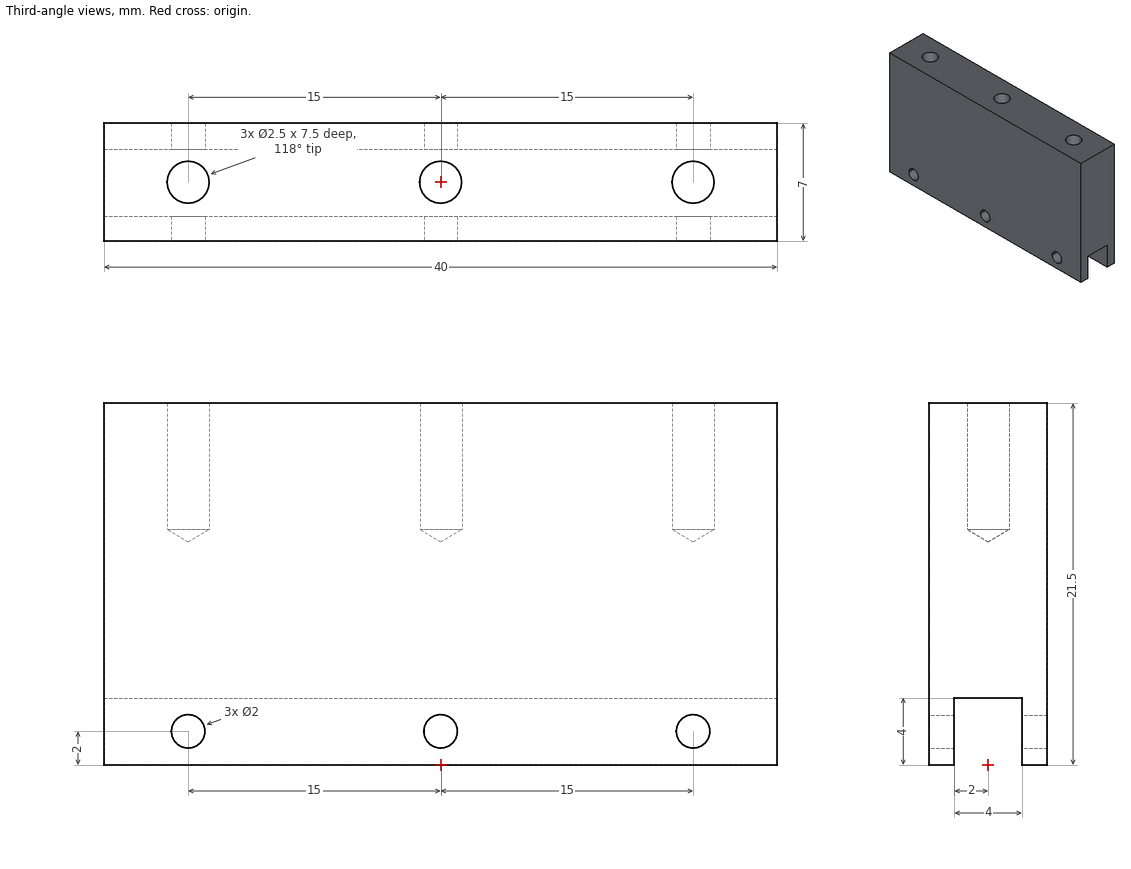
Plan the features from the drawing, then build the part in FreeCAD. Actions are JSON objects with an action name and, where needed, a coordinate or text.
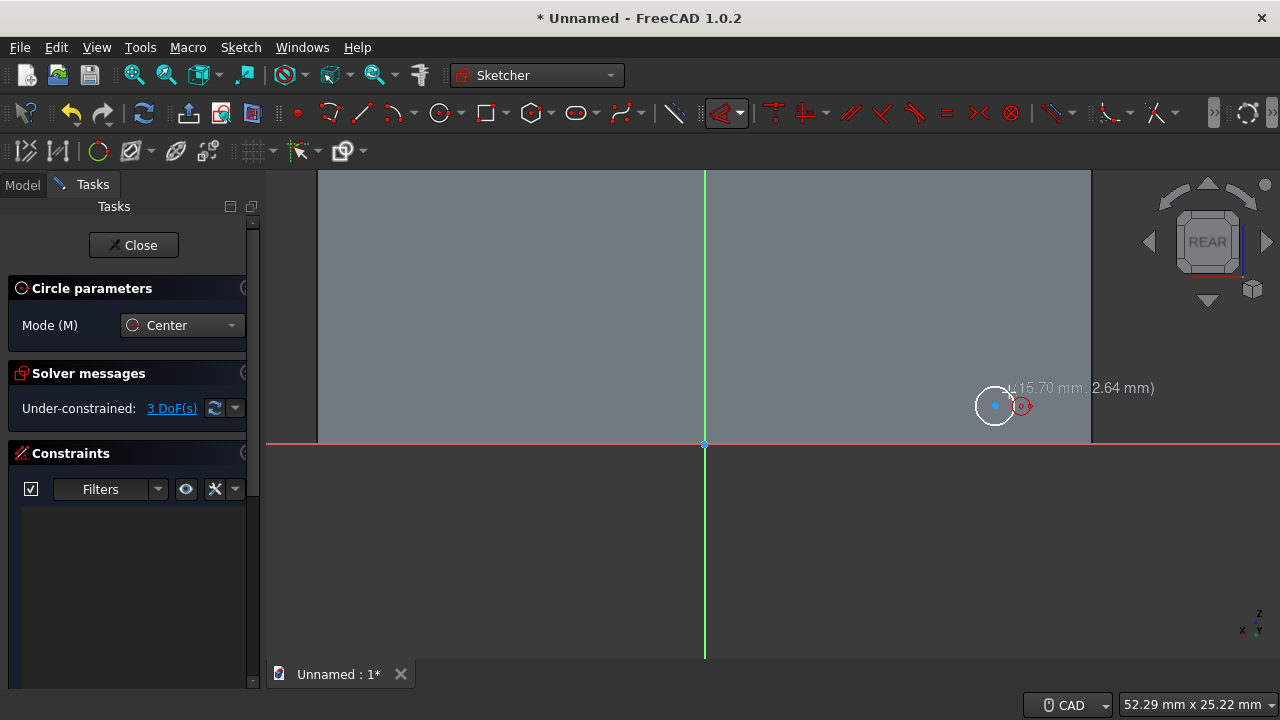
{"action": "left_click", "coordinate": [705, 405]}
{"action": "left_click", "coordinate": [723, 399]}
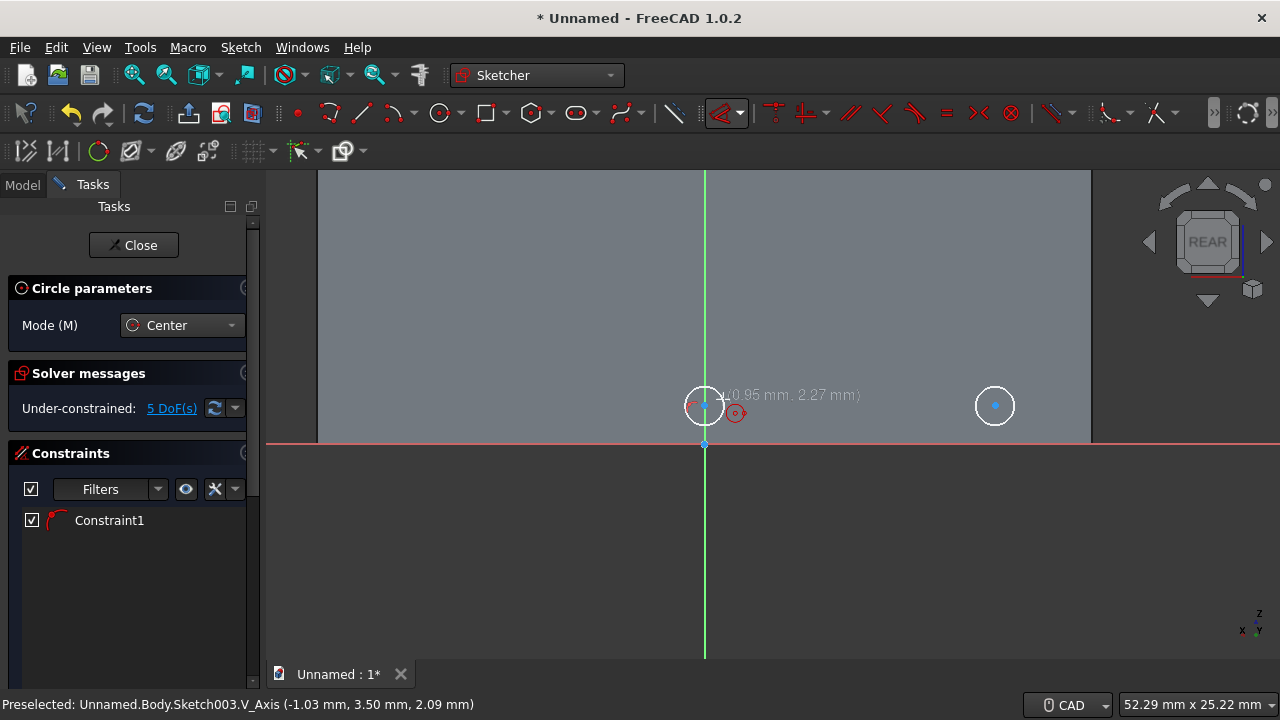
{"action": "left_click", "coordinate": [414, 405]}
{"action": "left_click", "coordinate": [427, 392]}
{"action": "key", "text": "Escape"}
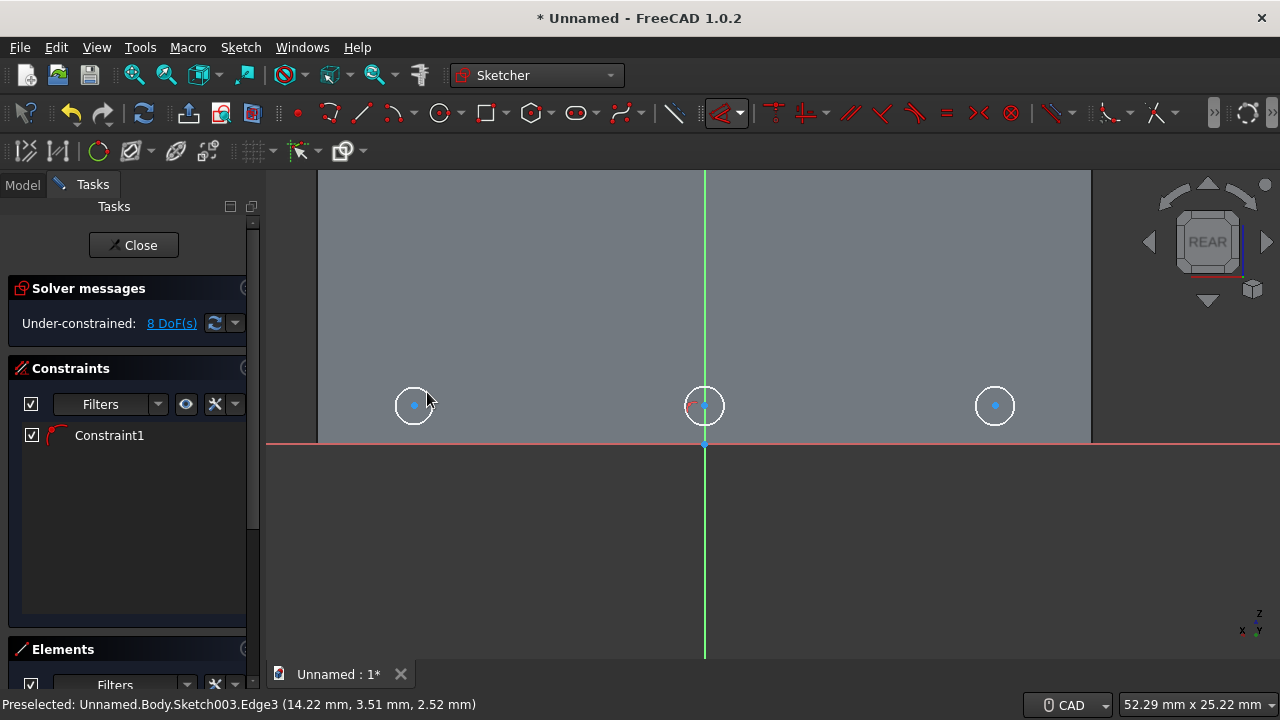
{"action": "left_click", "coordinate": [1008, 392]}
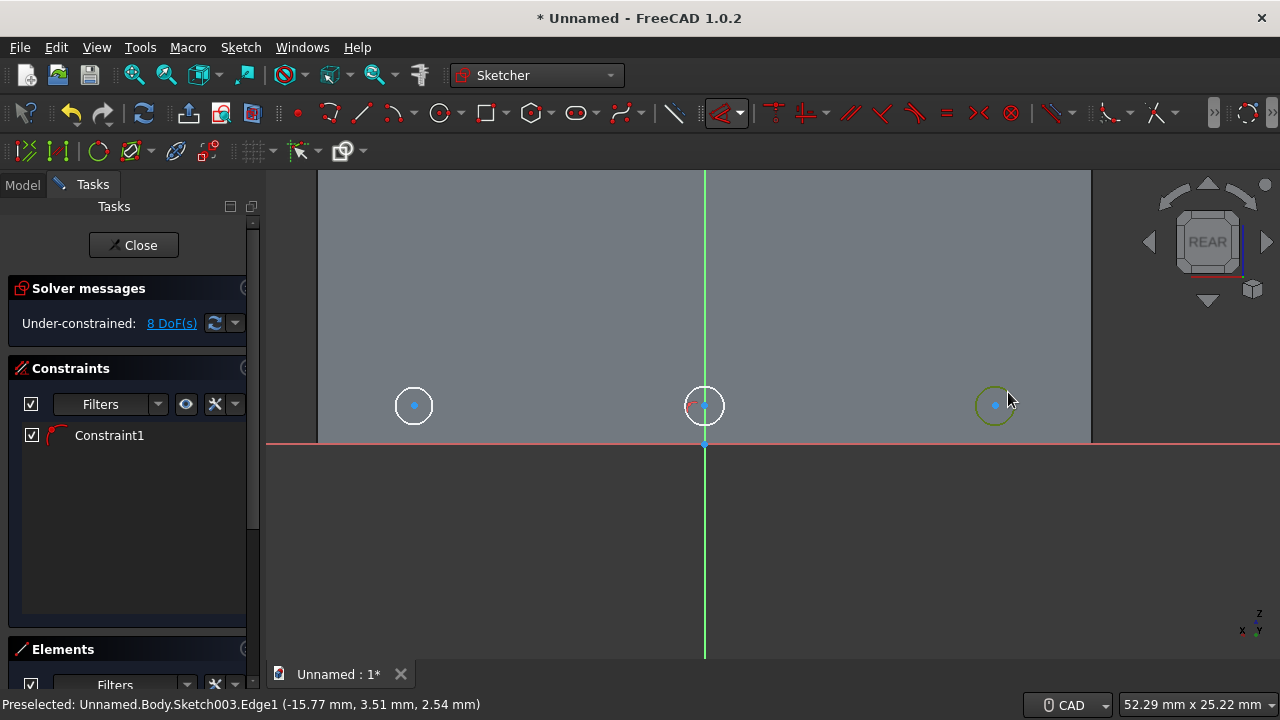
{"action": "left_click", "coordinate": [718, 392]}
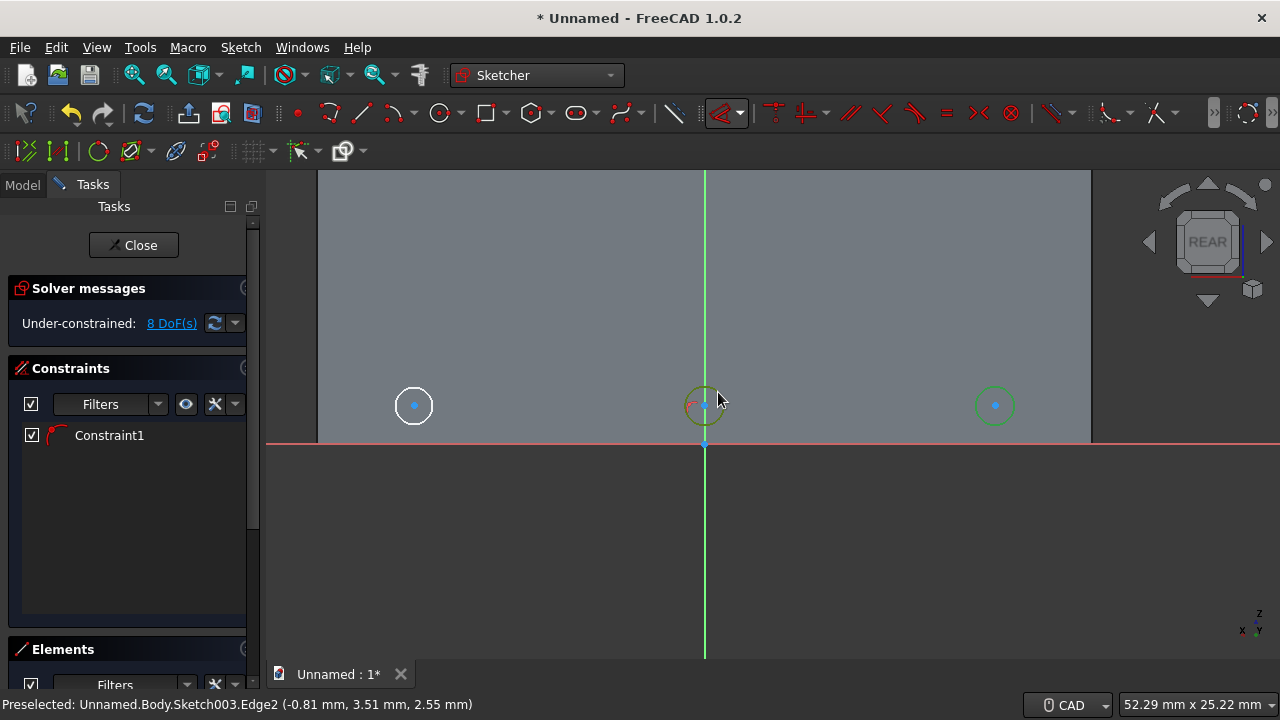
{"action": "left_click", "coordinate": [427, 393]}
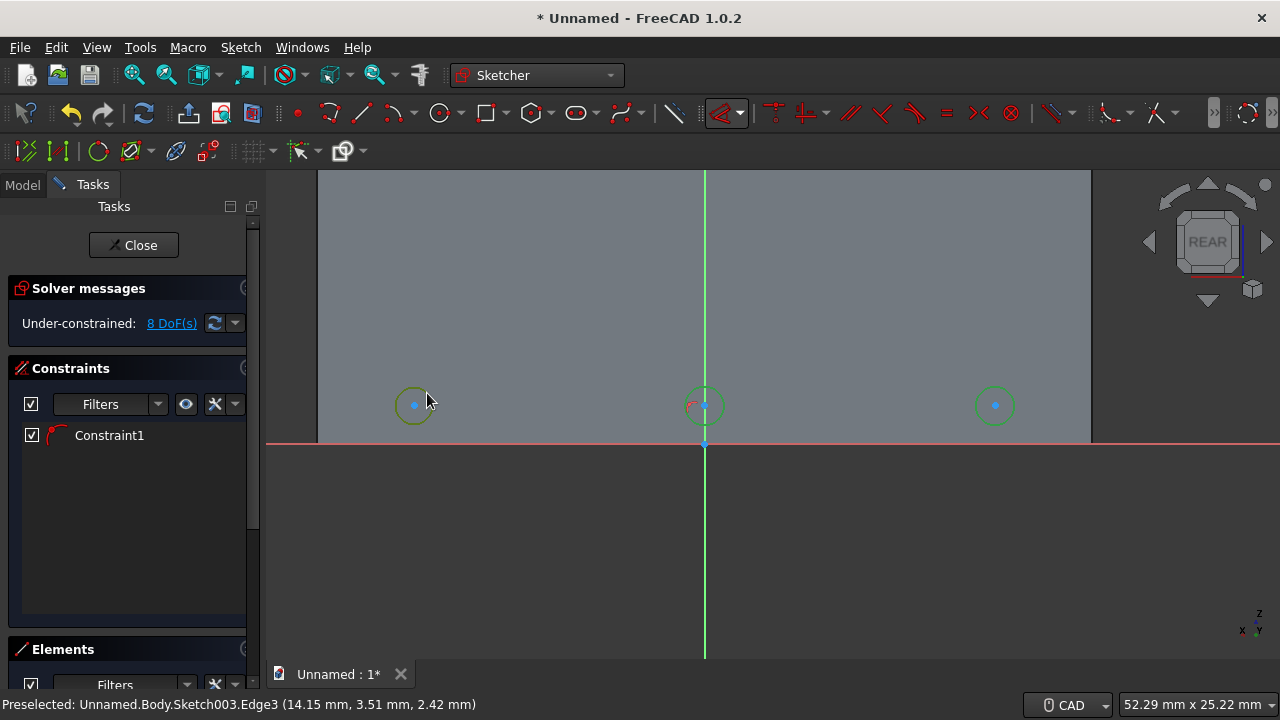
{"action": "left_click", "coordinate": [948, 114]}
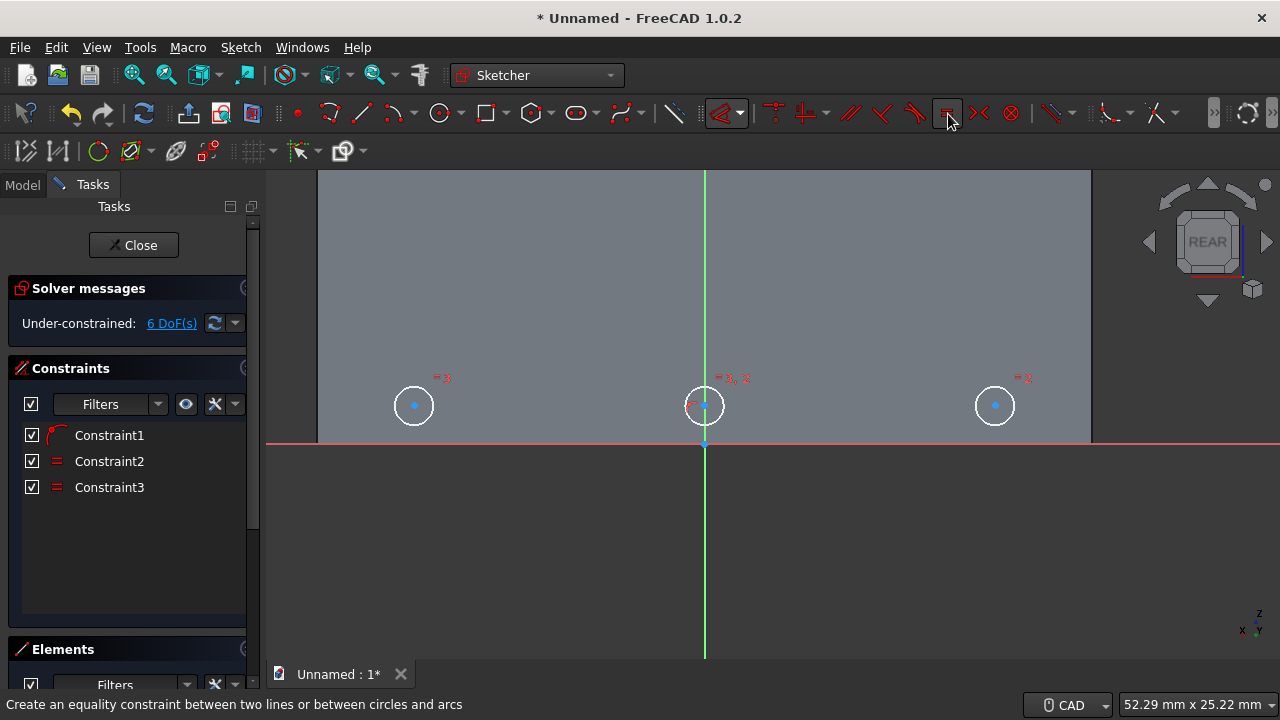
{"action": "left_click", "coordinate": [995, 406]}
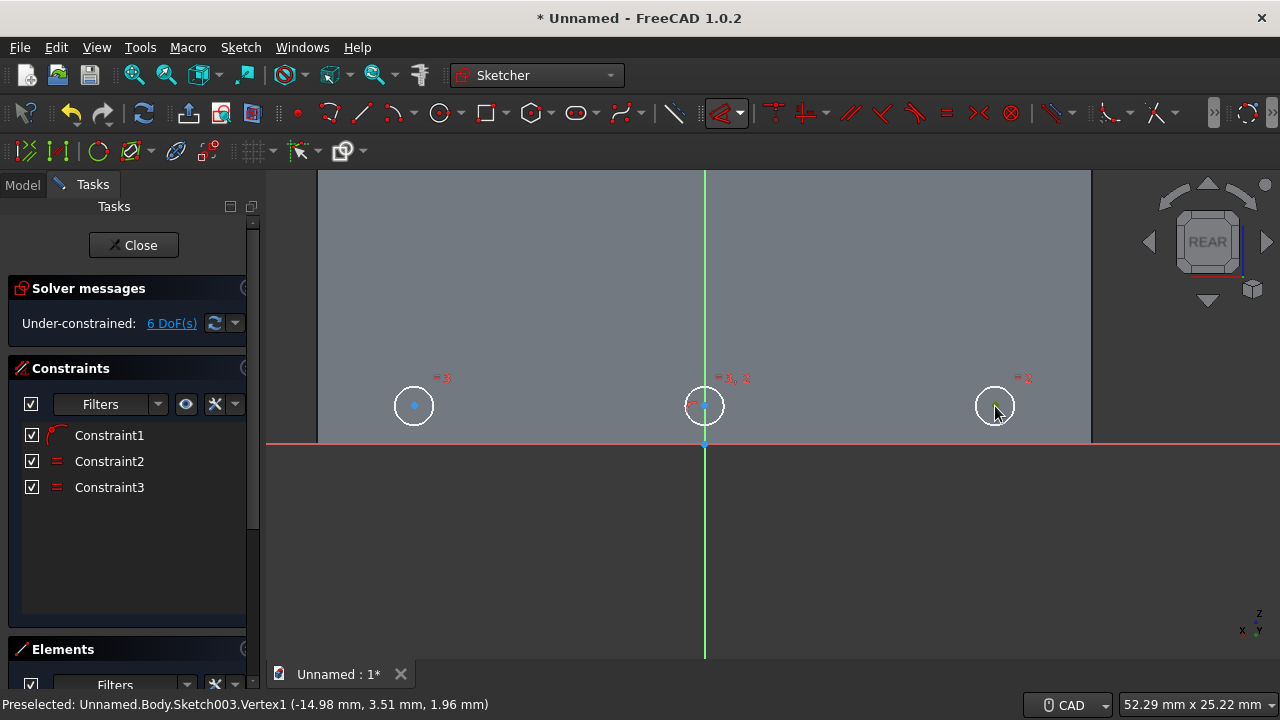
{"action": "left_click", "coordinate": [705, 406]}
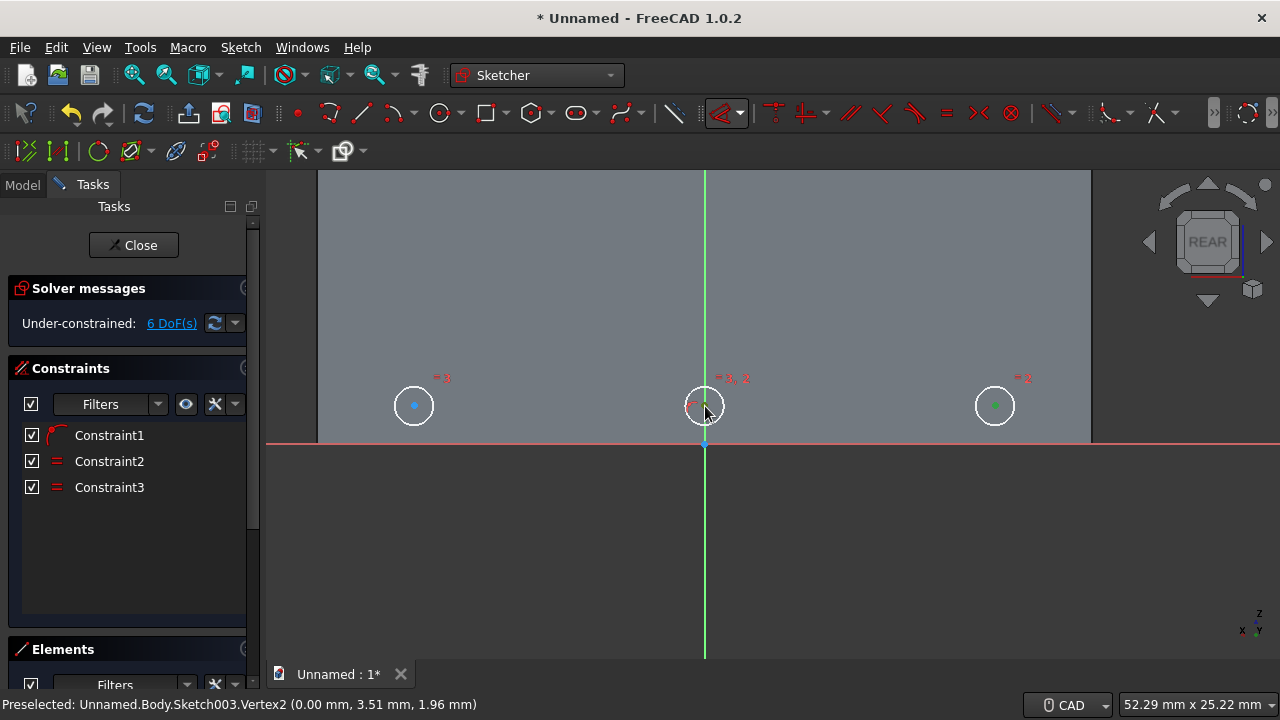
{"action": "left_click", "coordinate": [828, 114]}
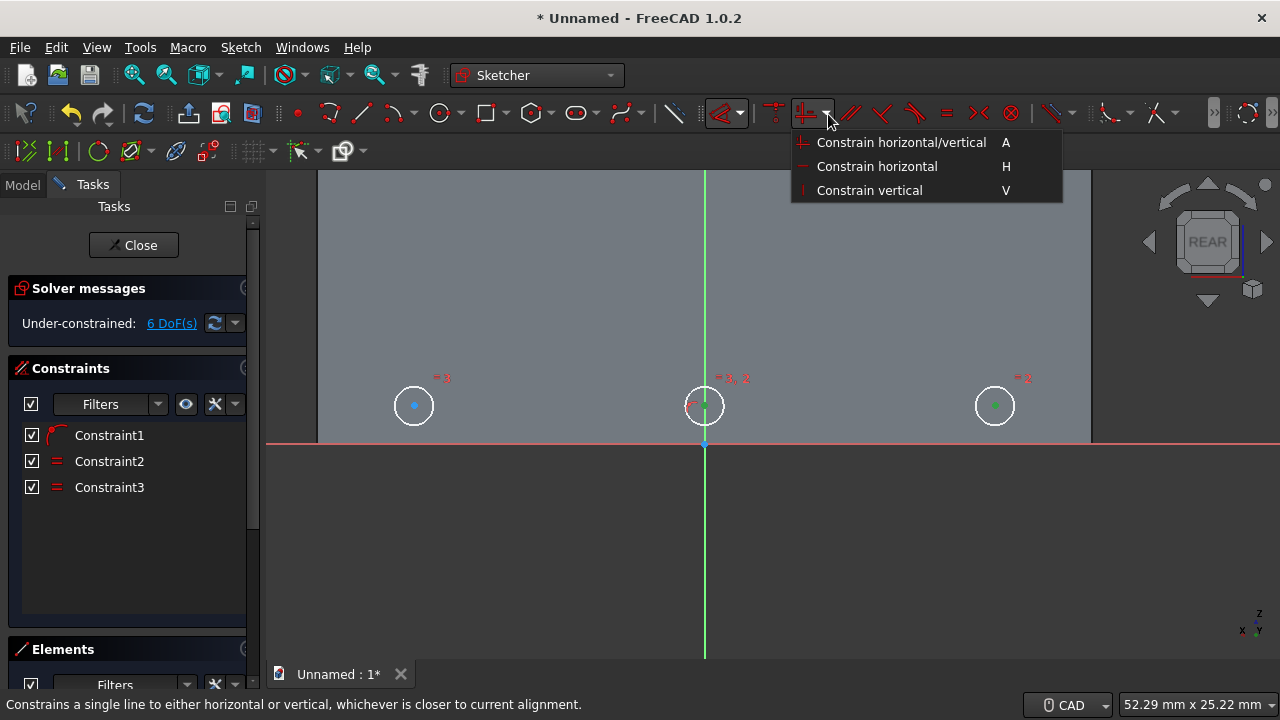
{"action": "left_click", "coordinate": [927, 166]}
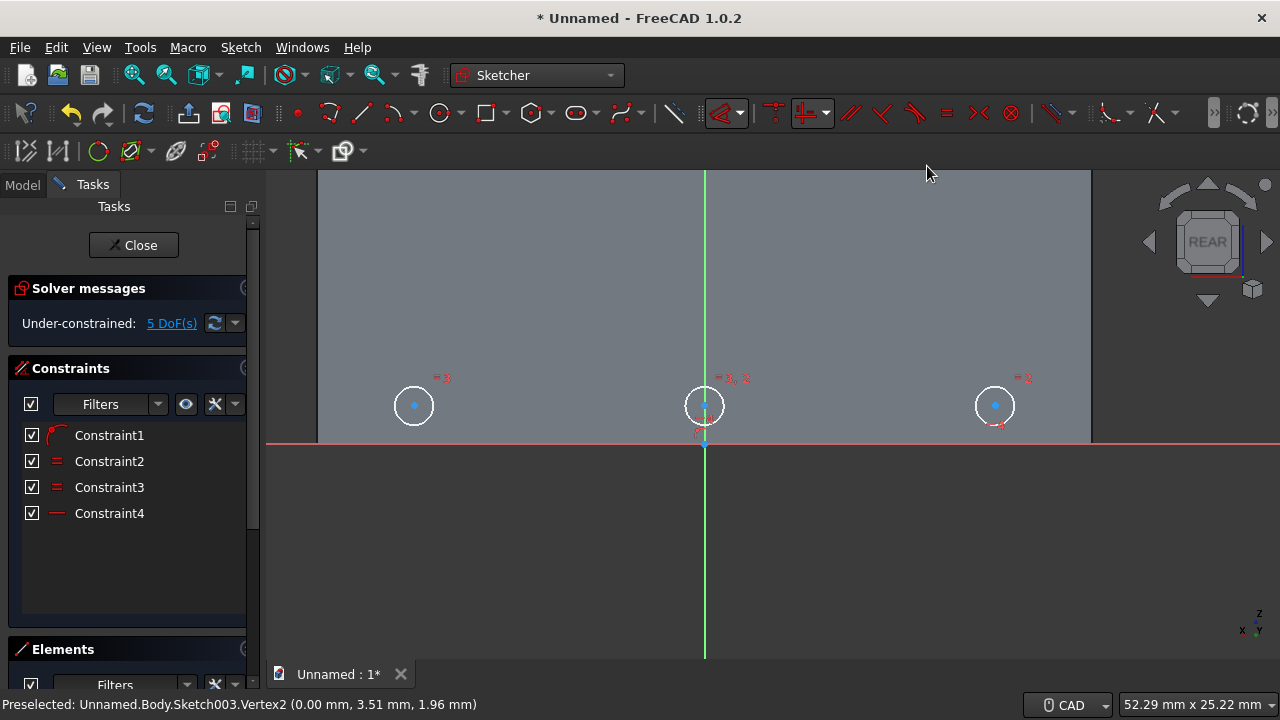
{"action": "left_click", "coordinate": [705, 406]}